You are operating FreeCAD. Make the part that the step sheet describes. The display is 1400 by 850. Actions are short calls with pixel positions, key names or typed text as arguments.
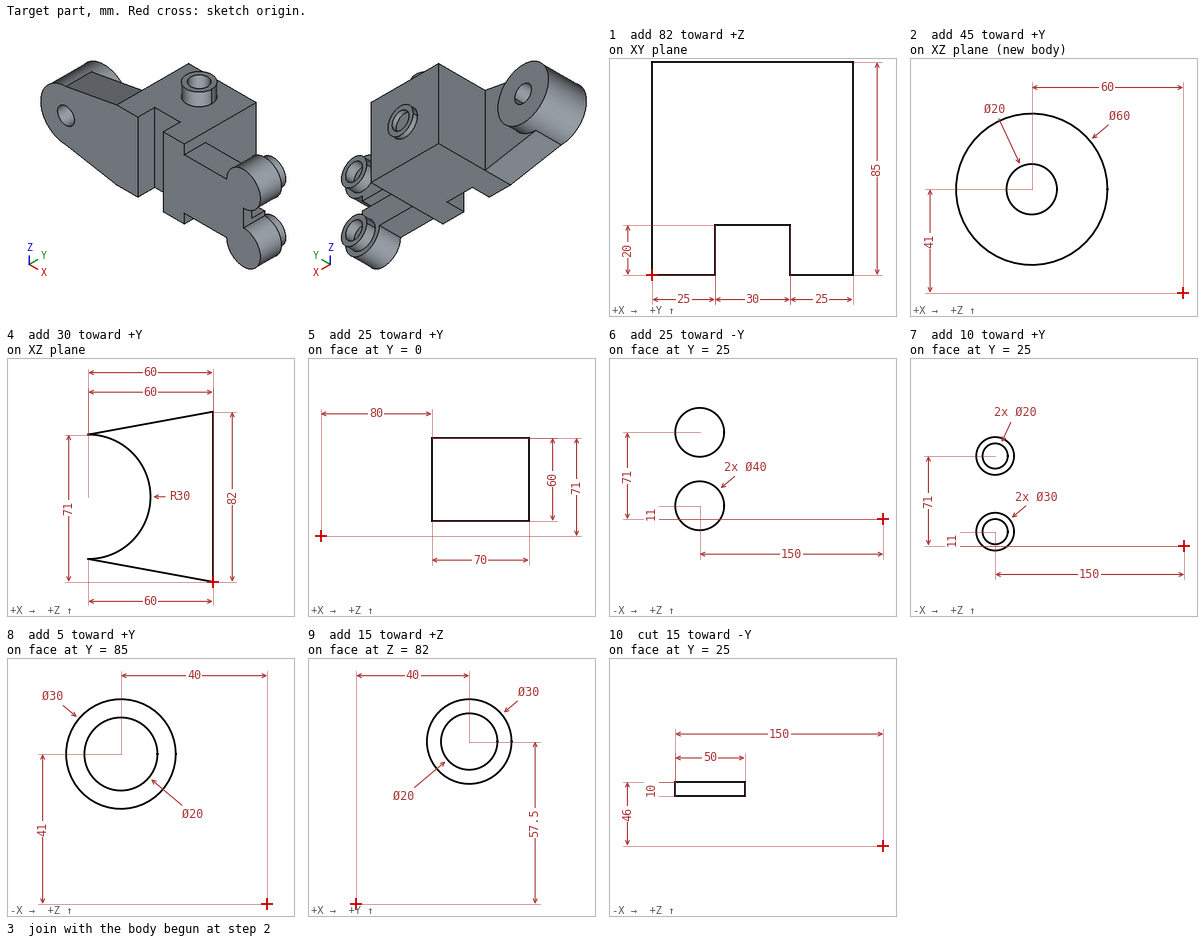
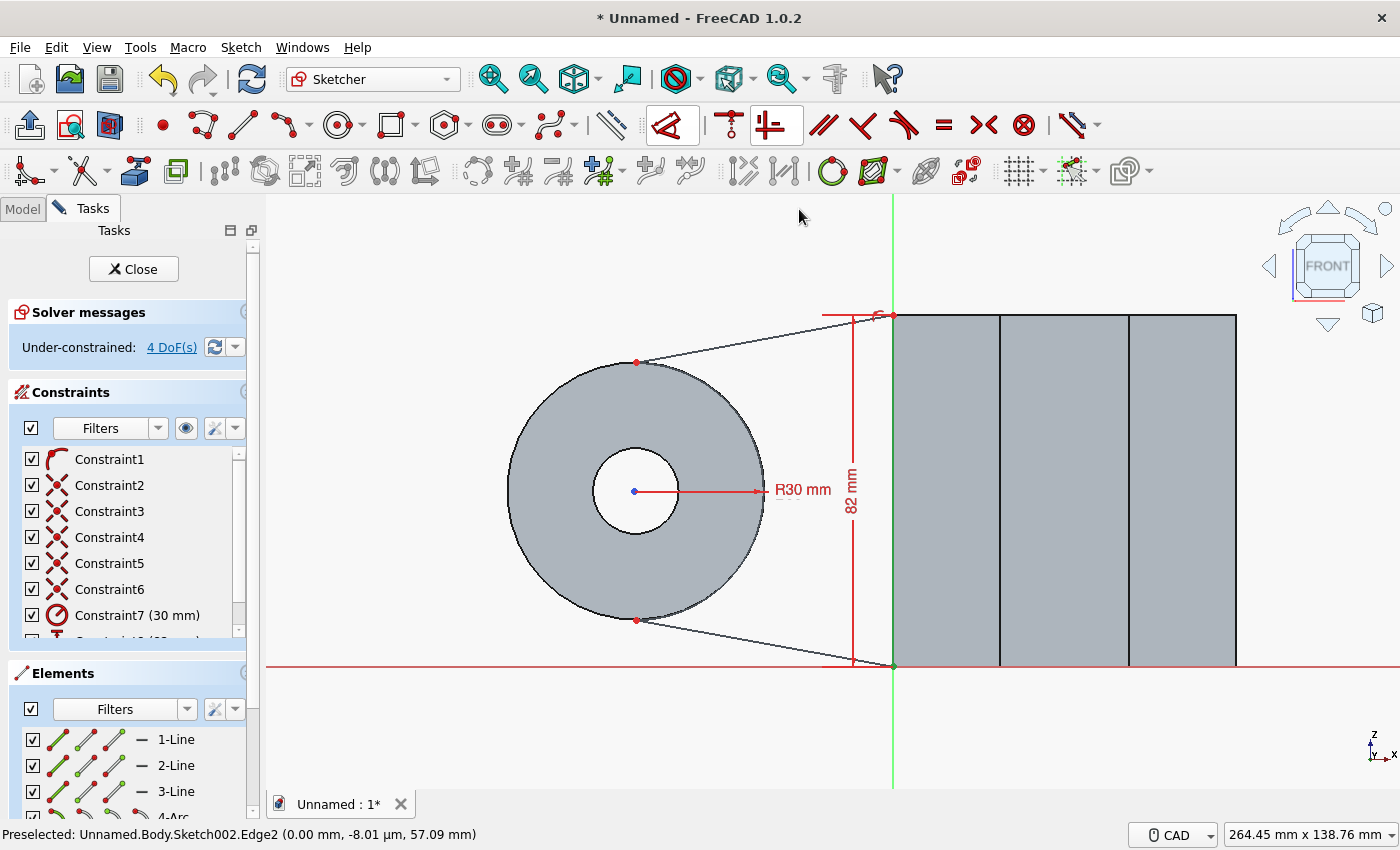
click(636, 363)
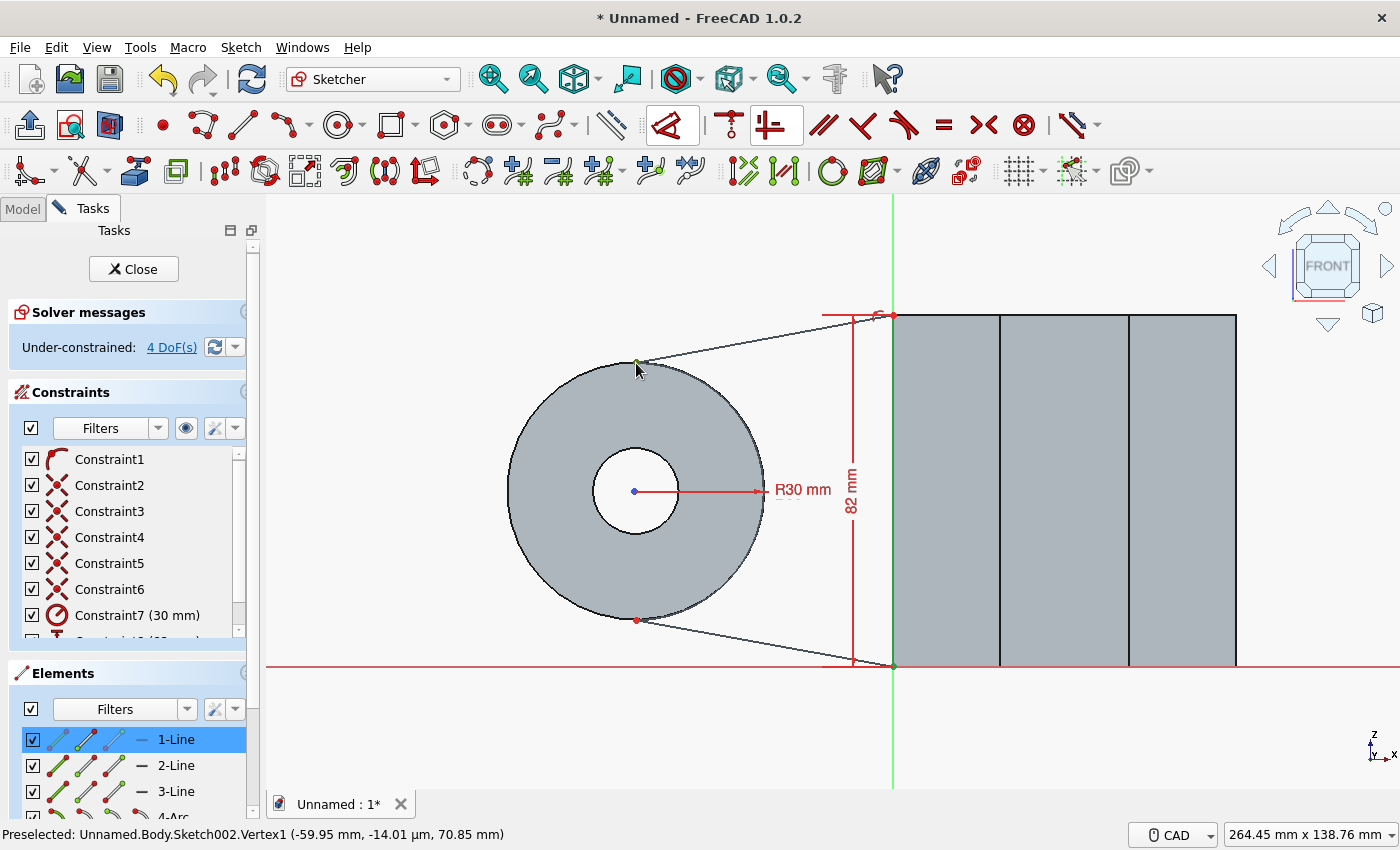
click(694, 126)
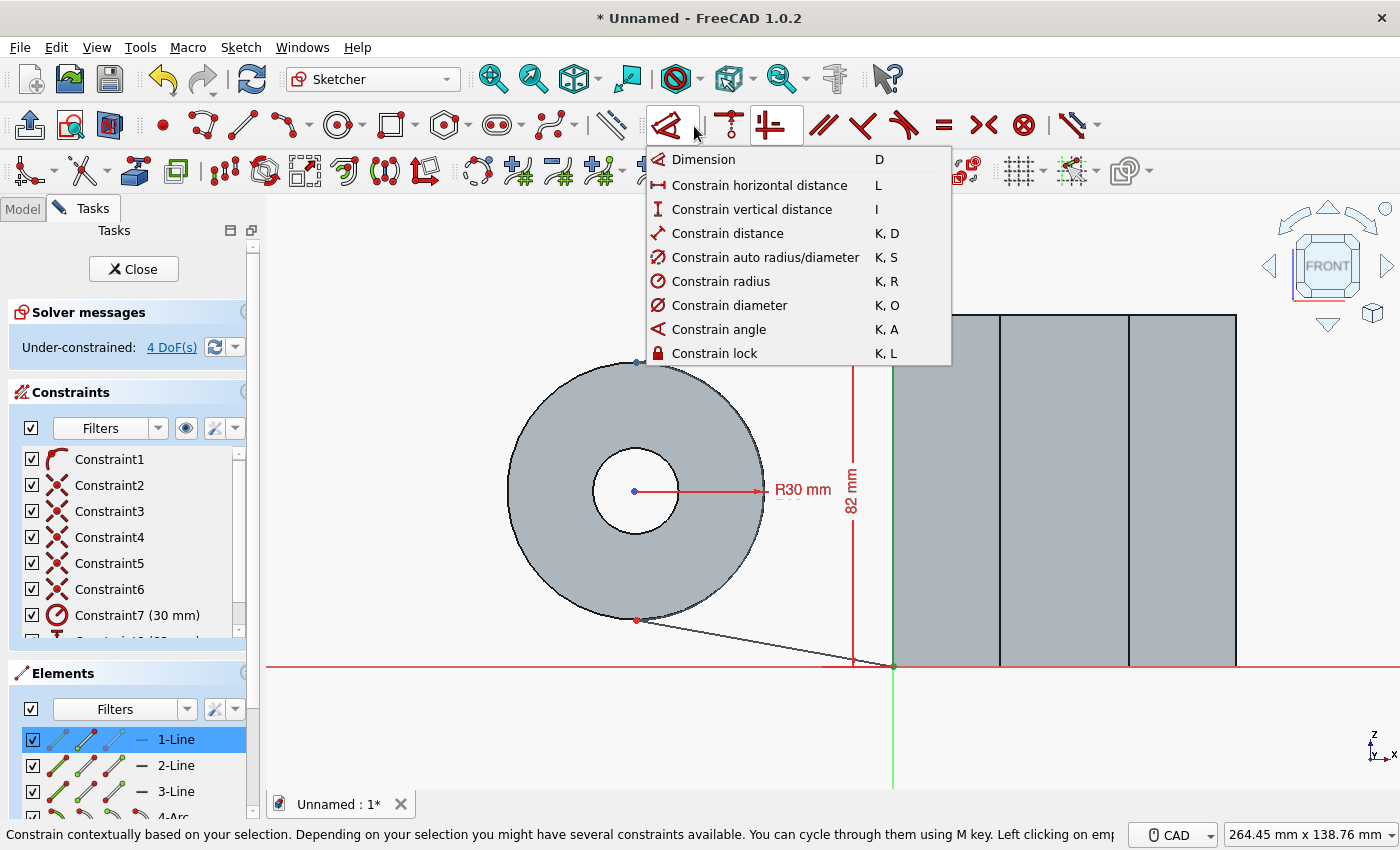
click(799, 185)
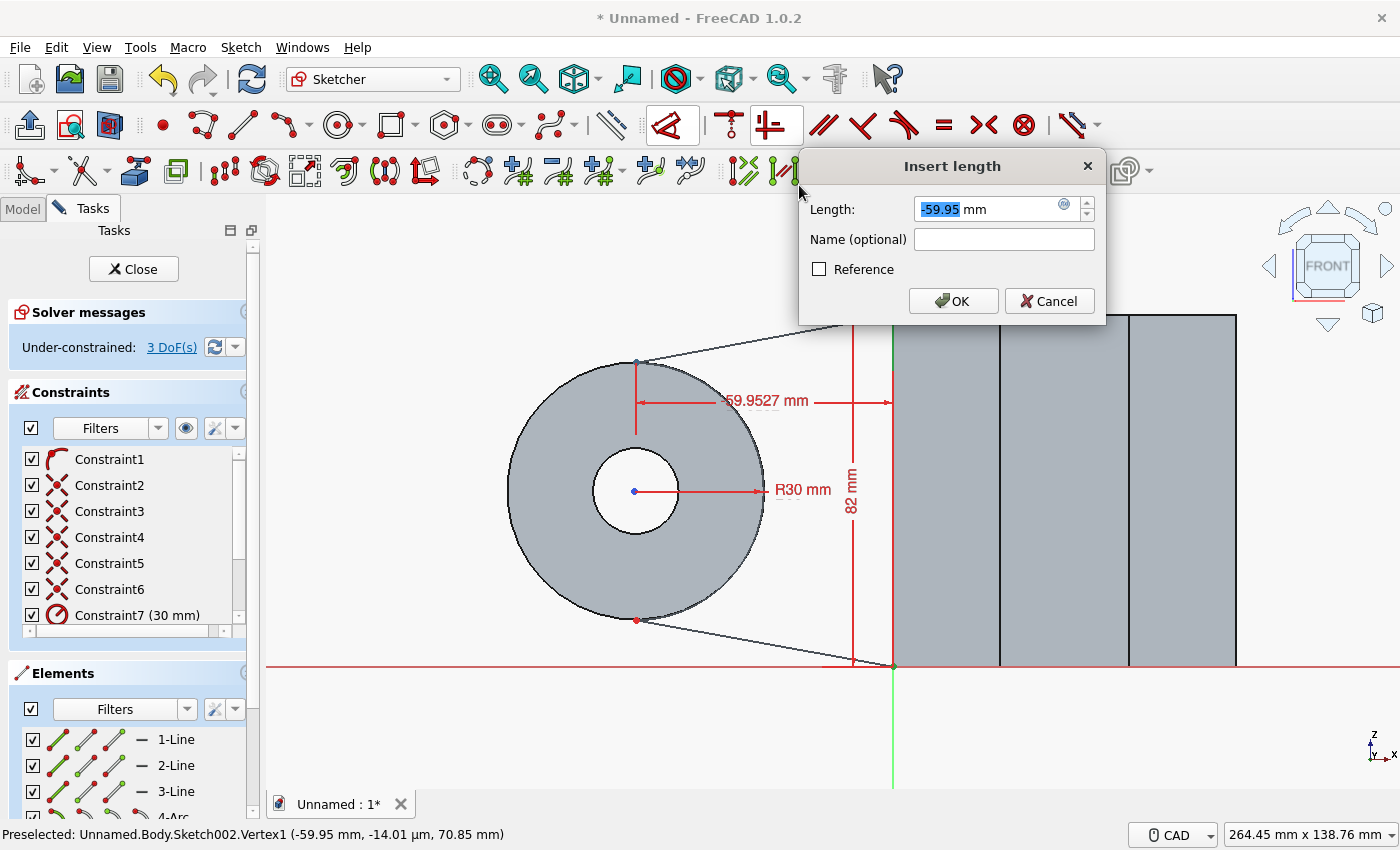
text(-60)
key(Return)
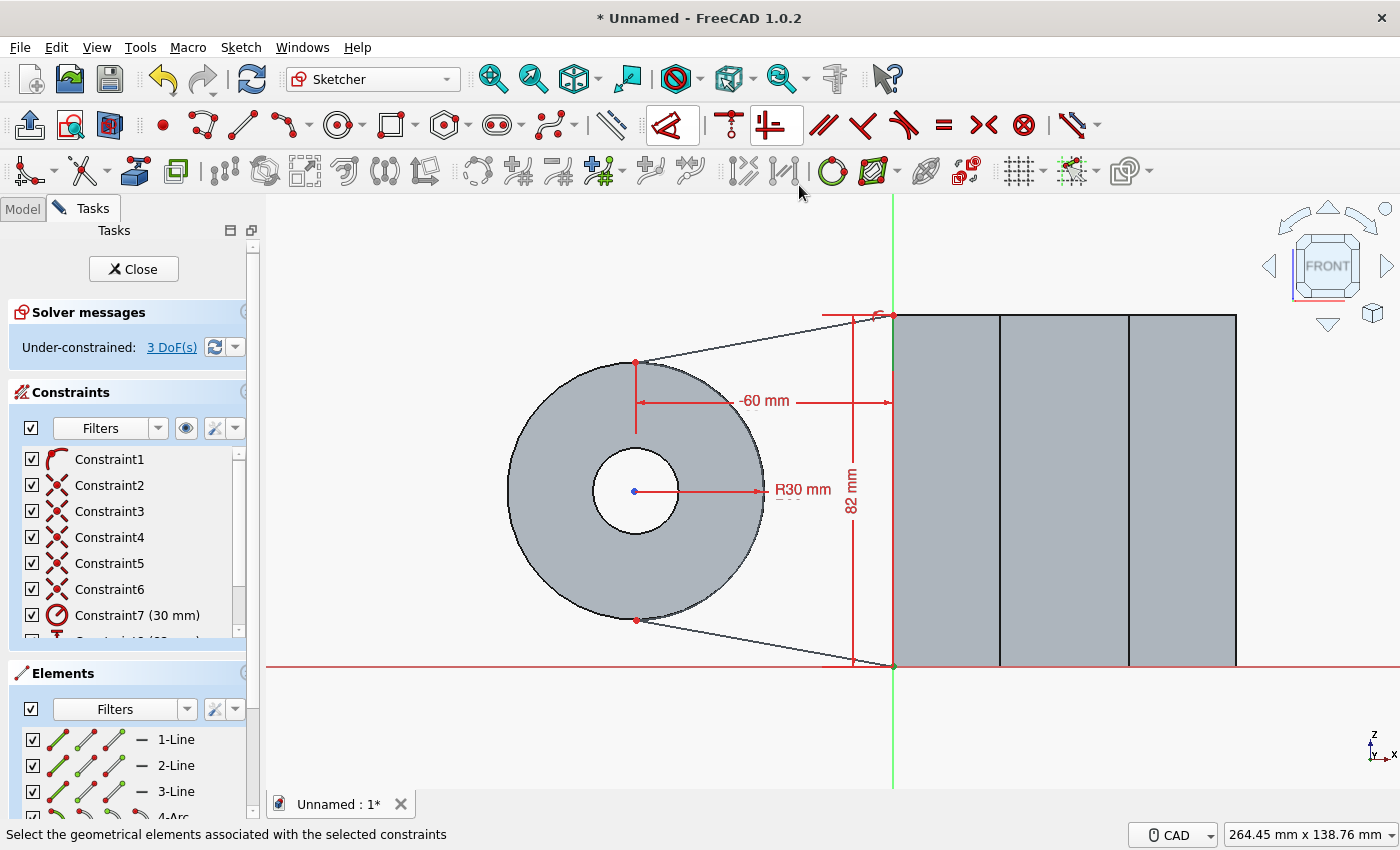
click(636, 363)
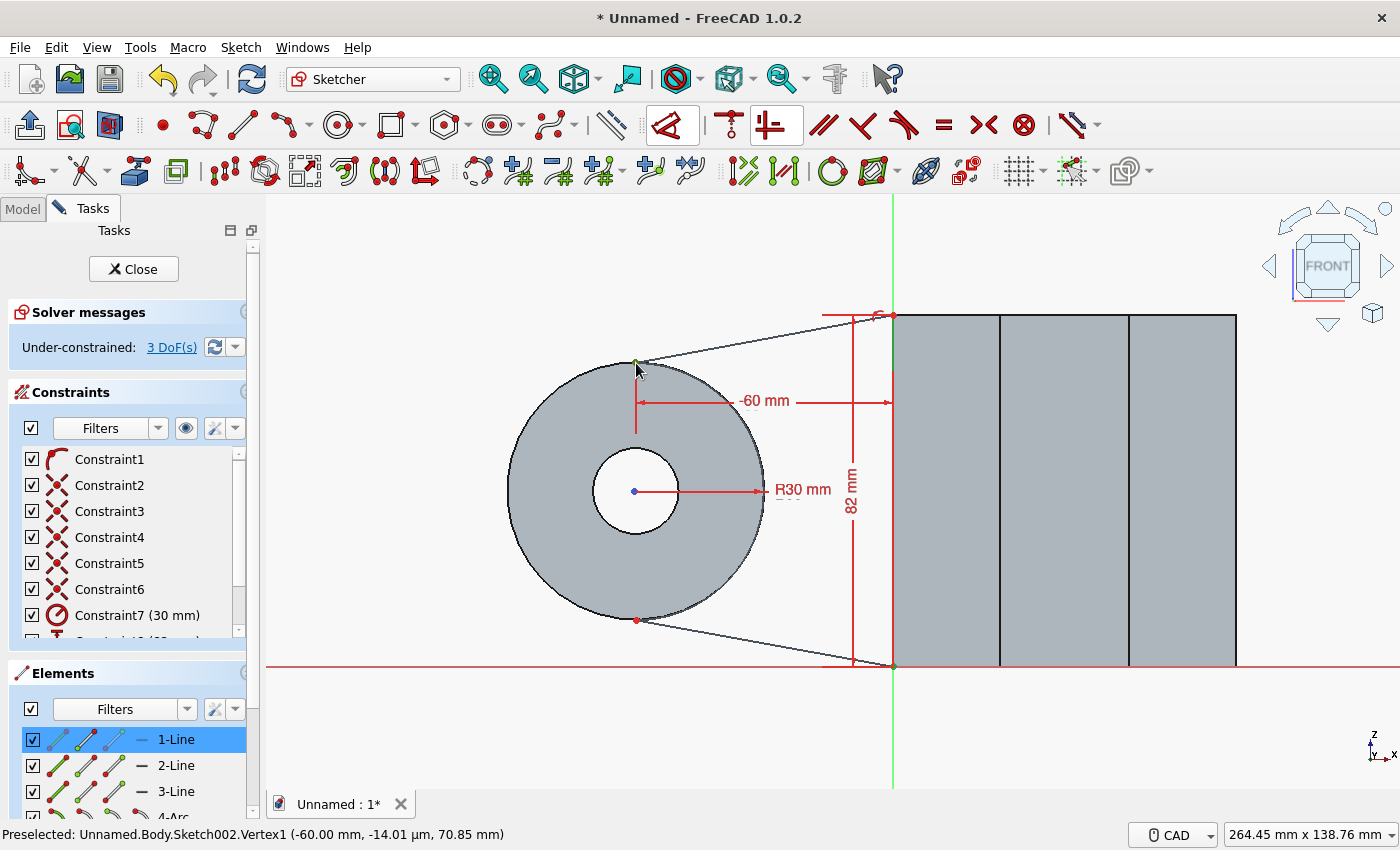
click(694, 126)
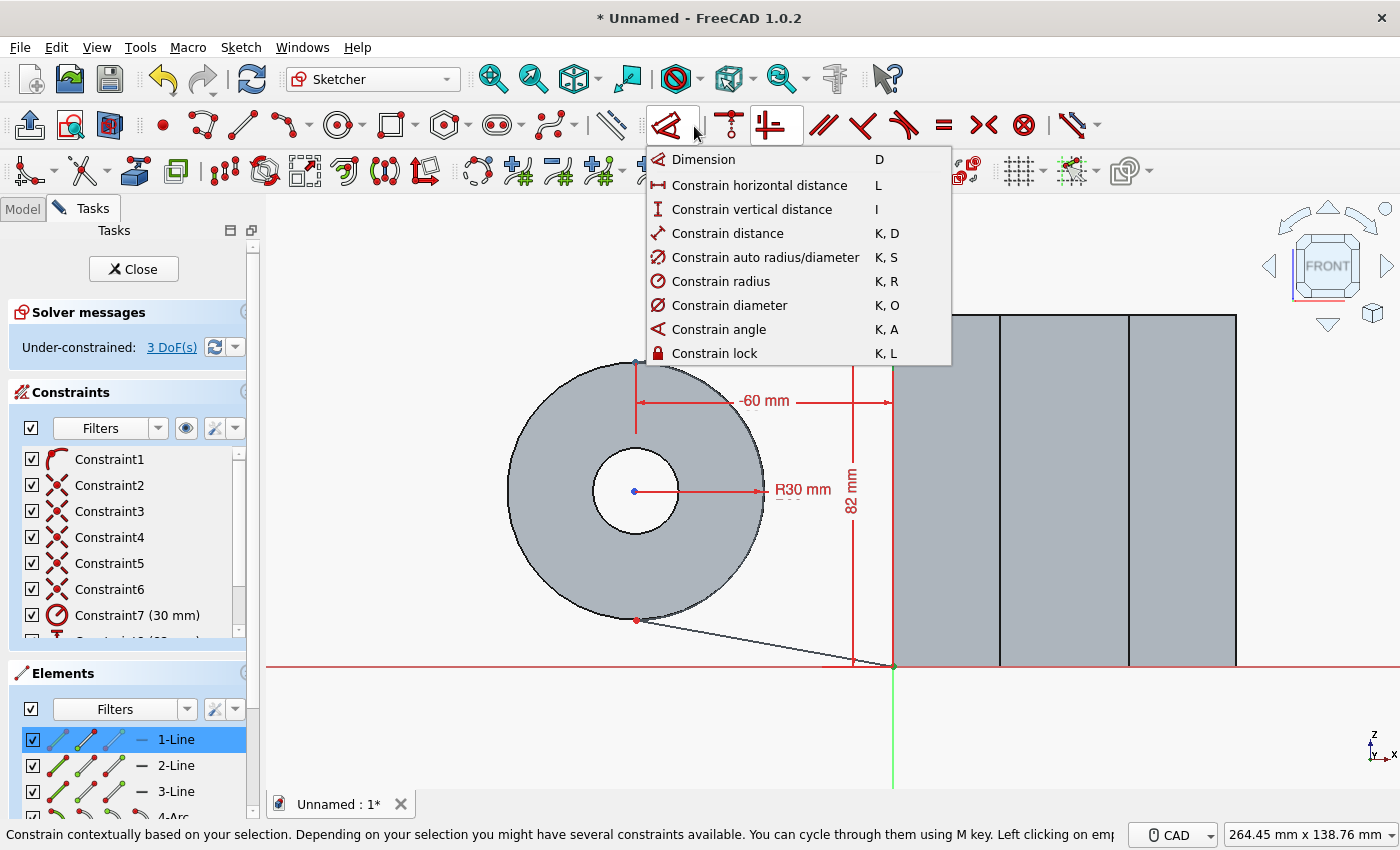
click(799, 209)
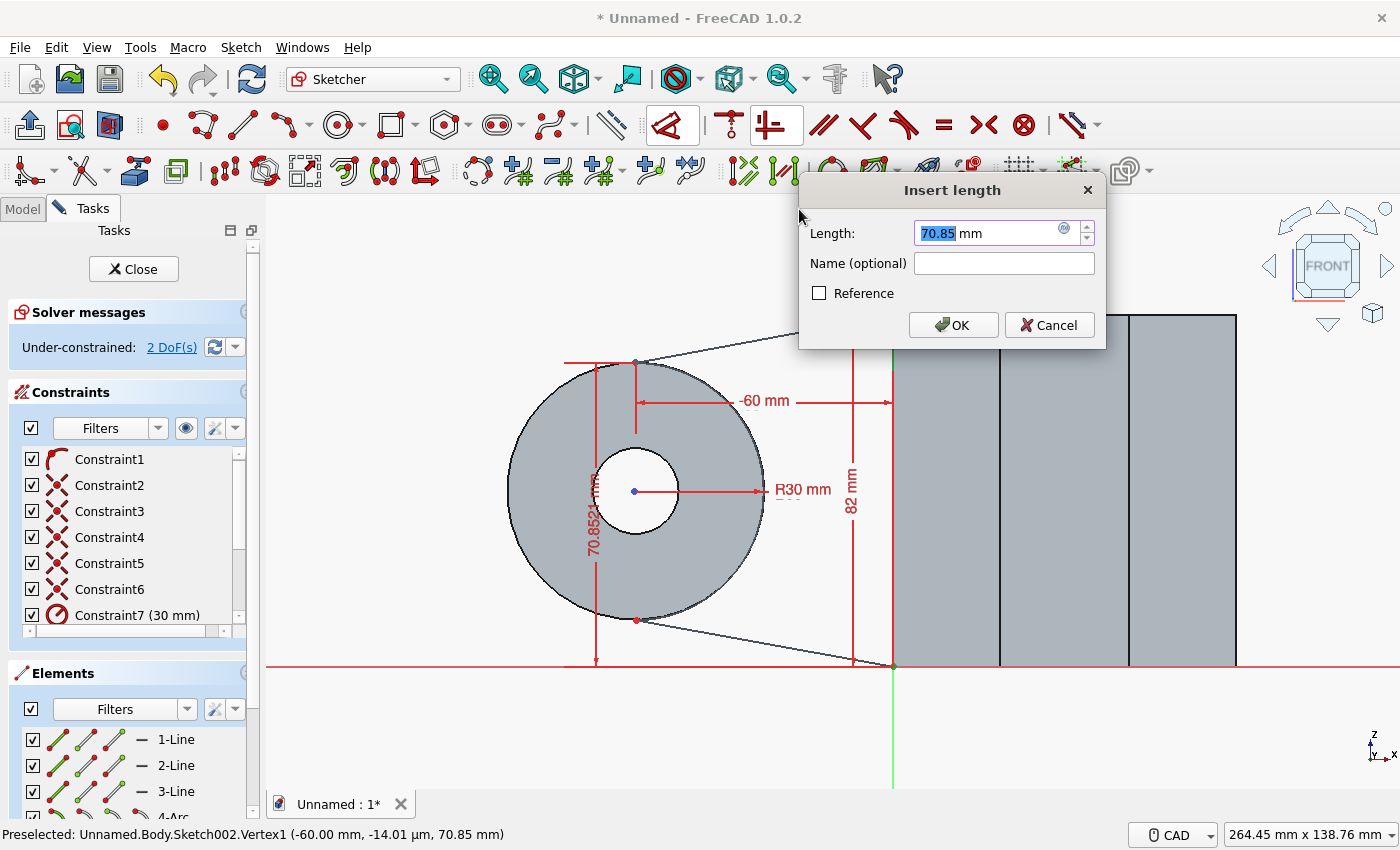
text(71)
key(Return)